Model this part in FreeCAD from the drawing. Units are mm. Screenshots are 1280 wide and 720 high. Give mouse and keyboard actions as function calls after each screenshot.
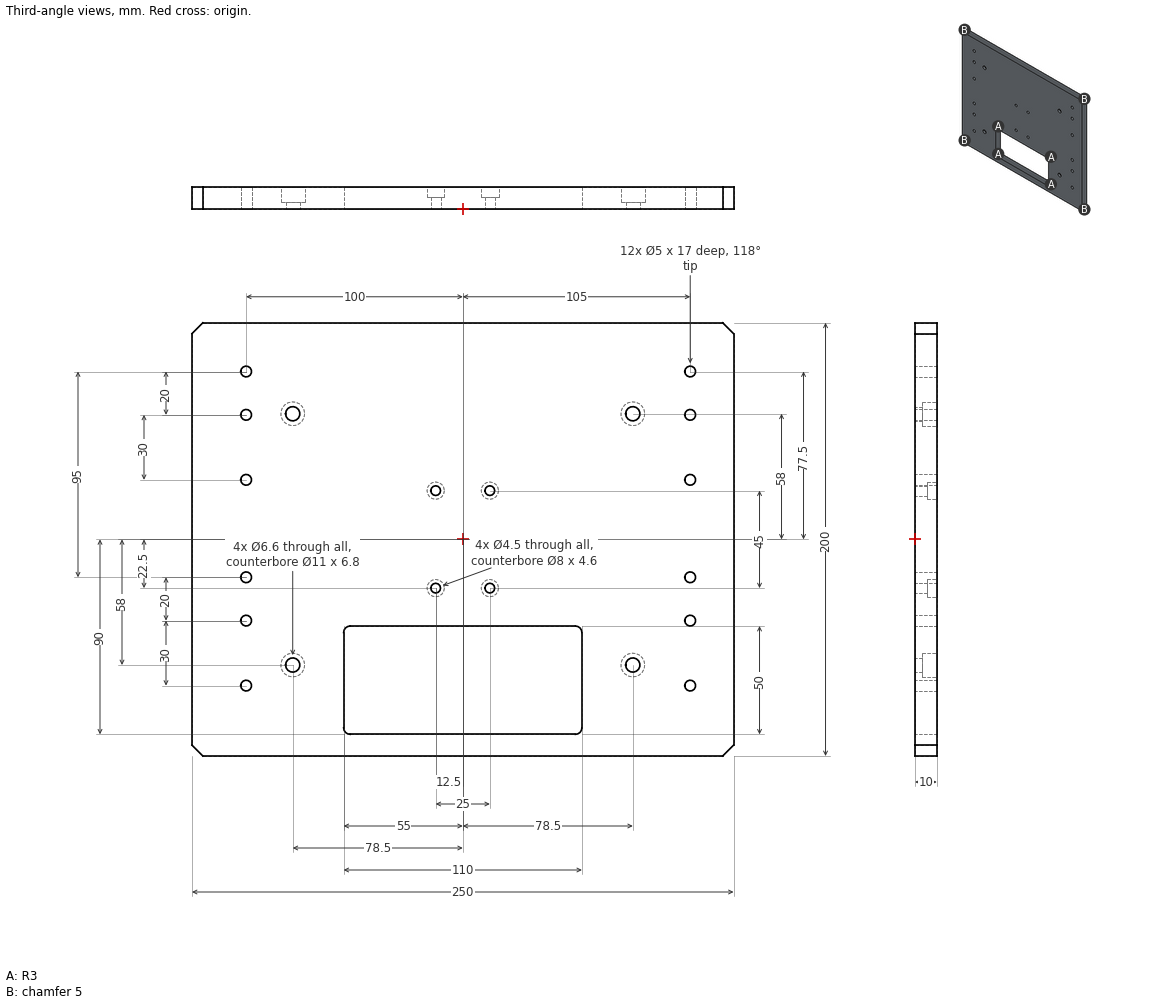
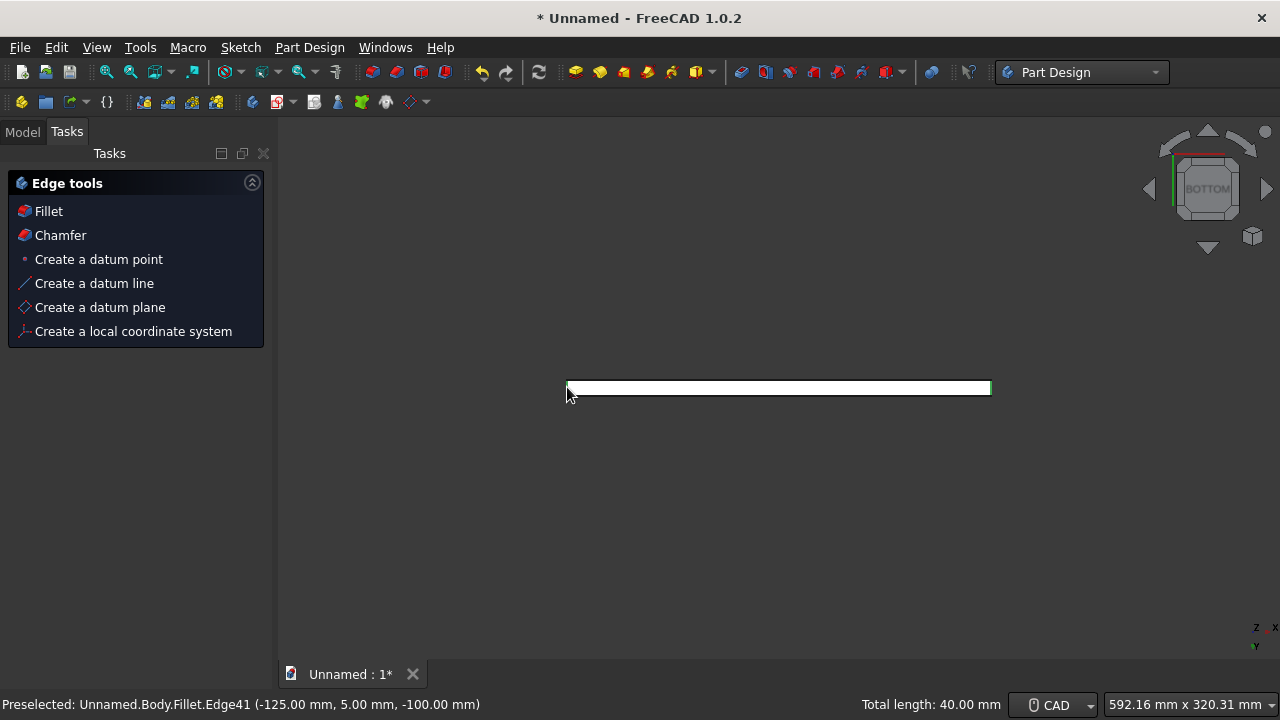
click(398, 72)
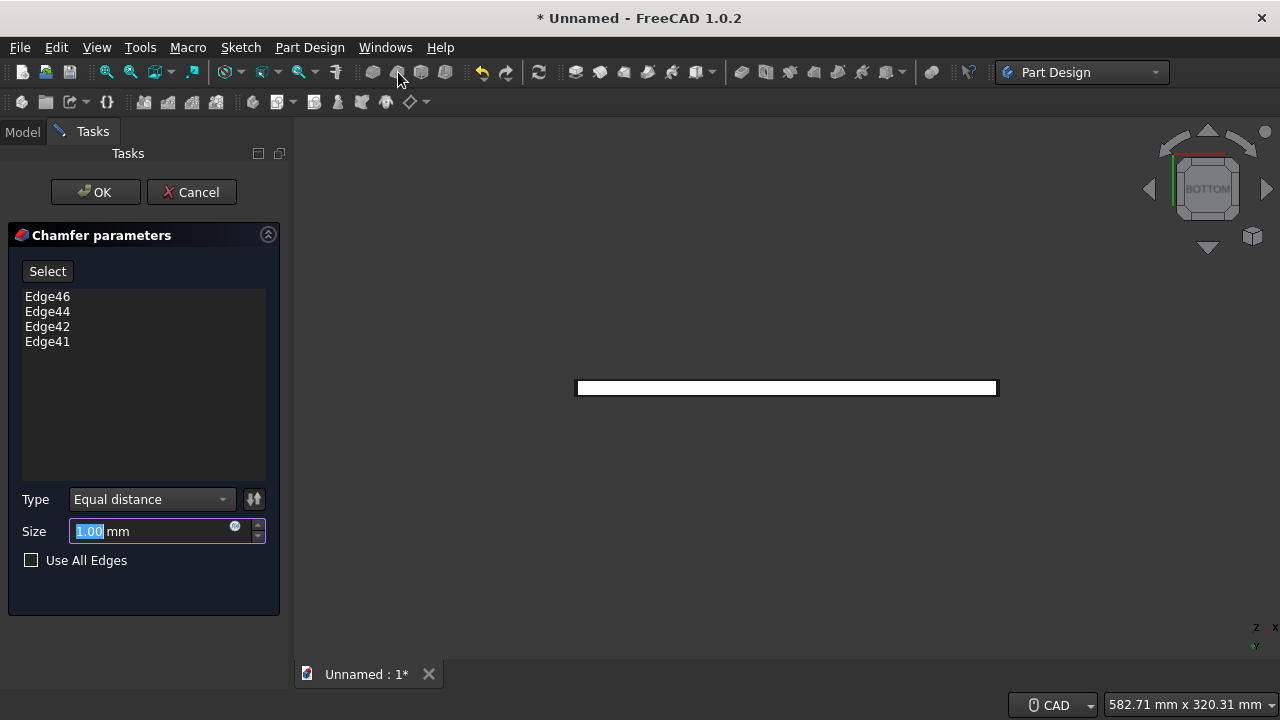
text(5)
key(Tab)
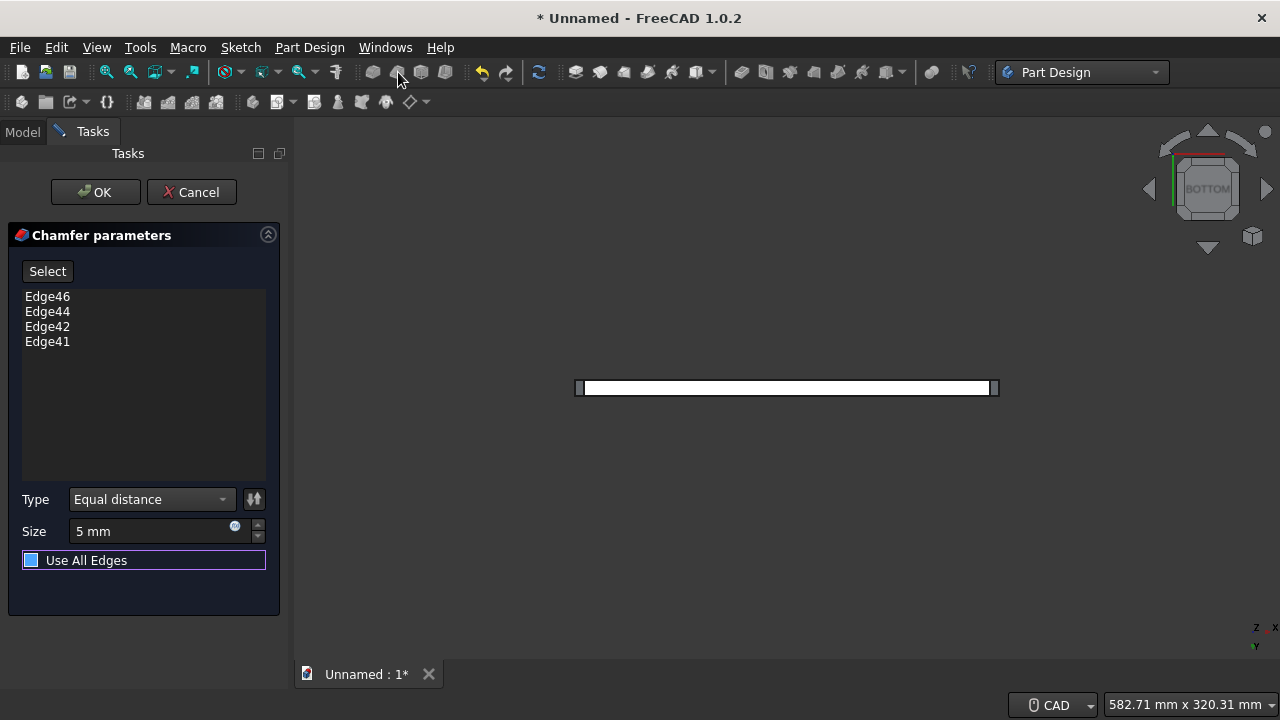
click(96, 192)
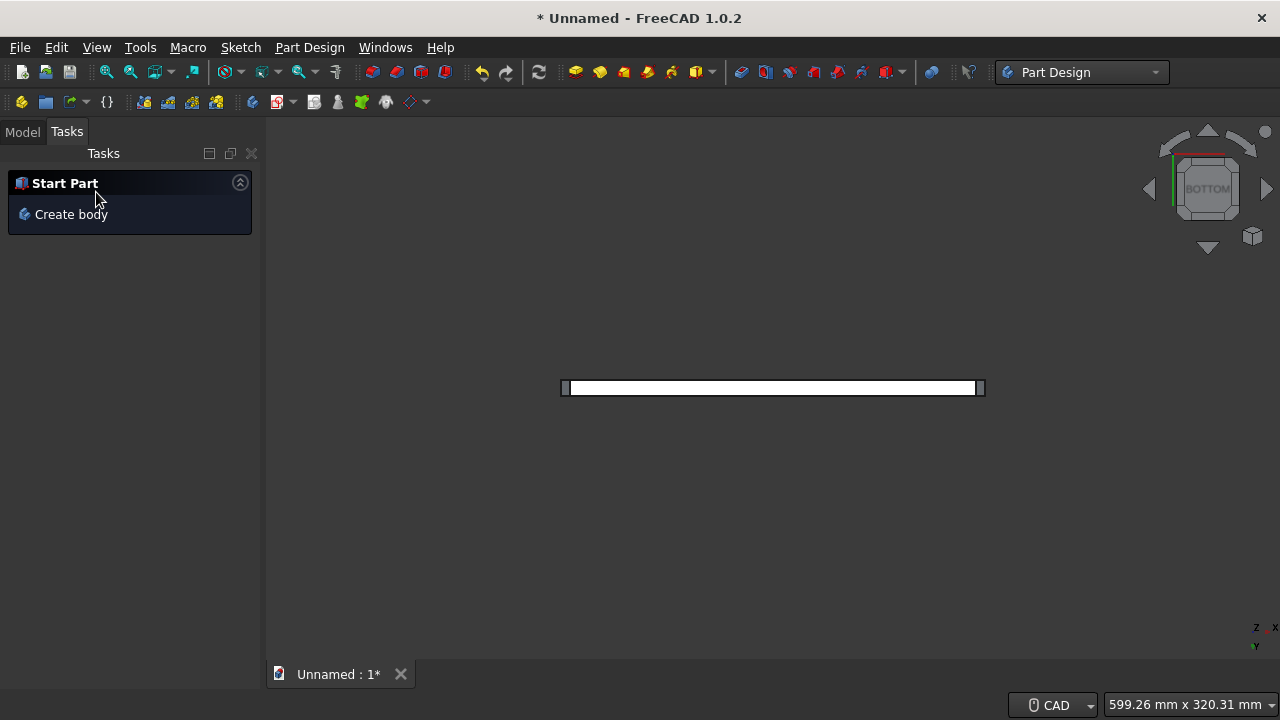
click(108, 72)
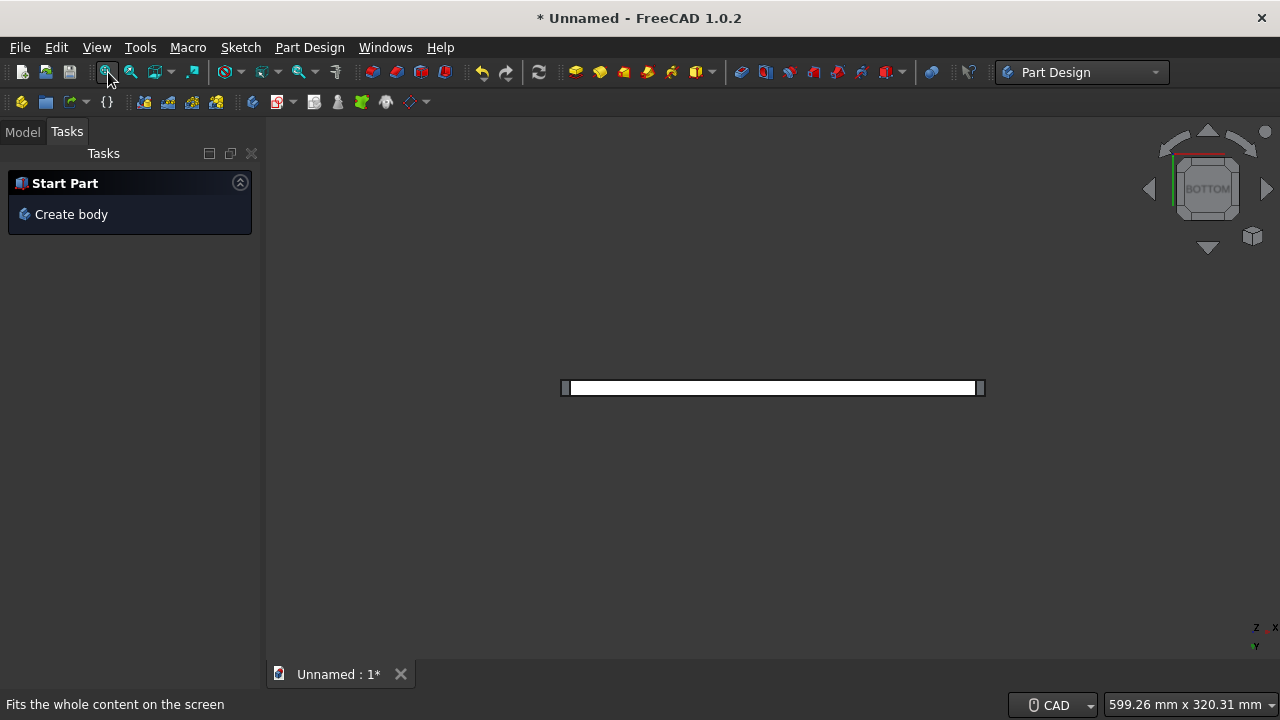
key(4)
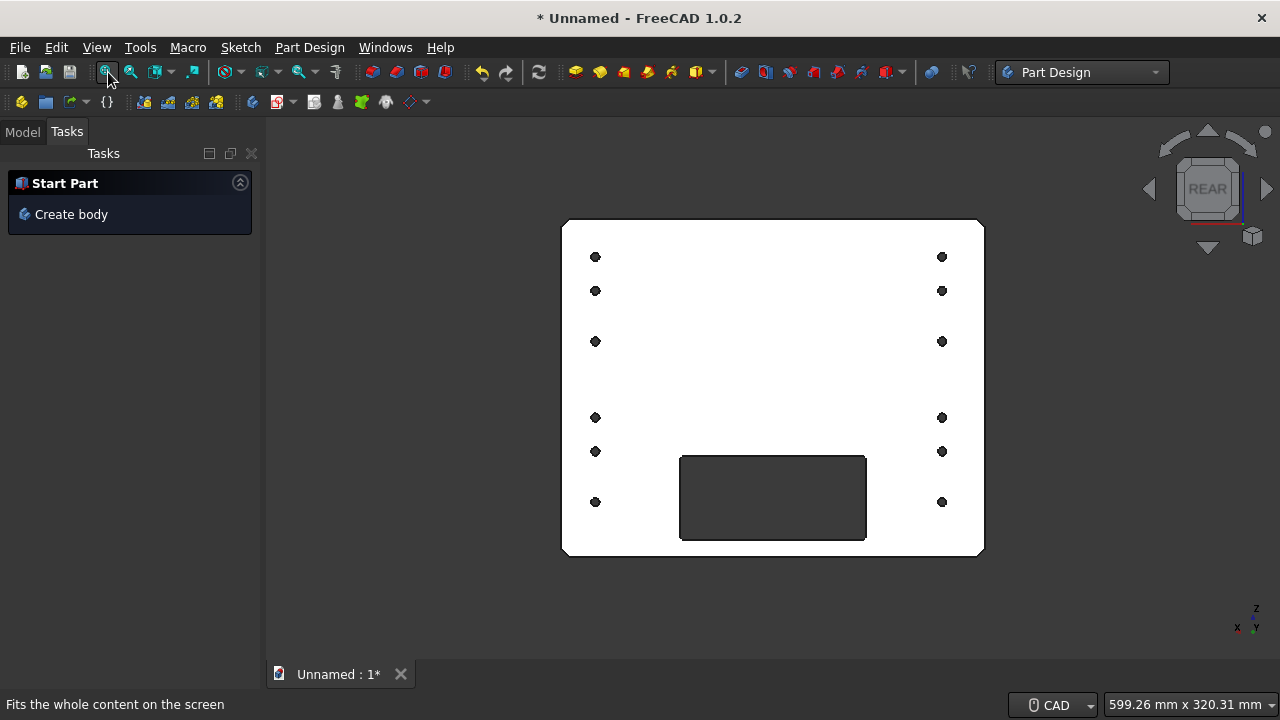
click(773, 339)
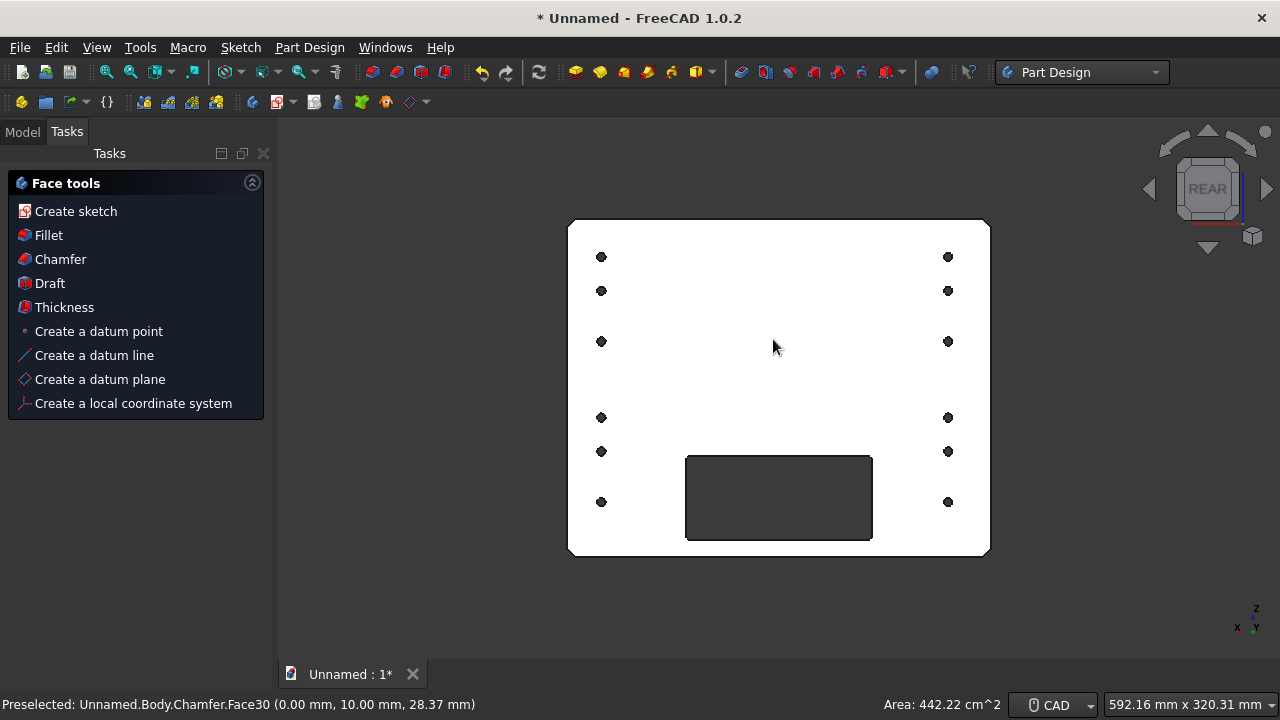
click(278, 102)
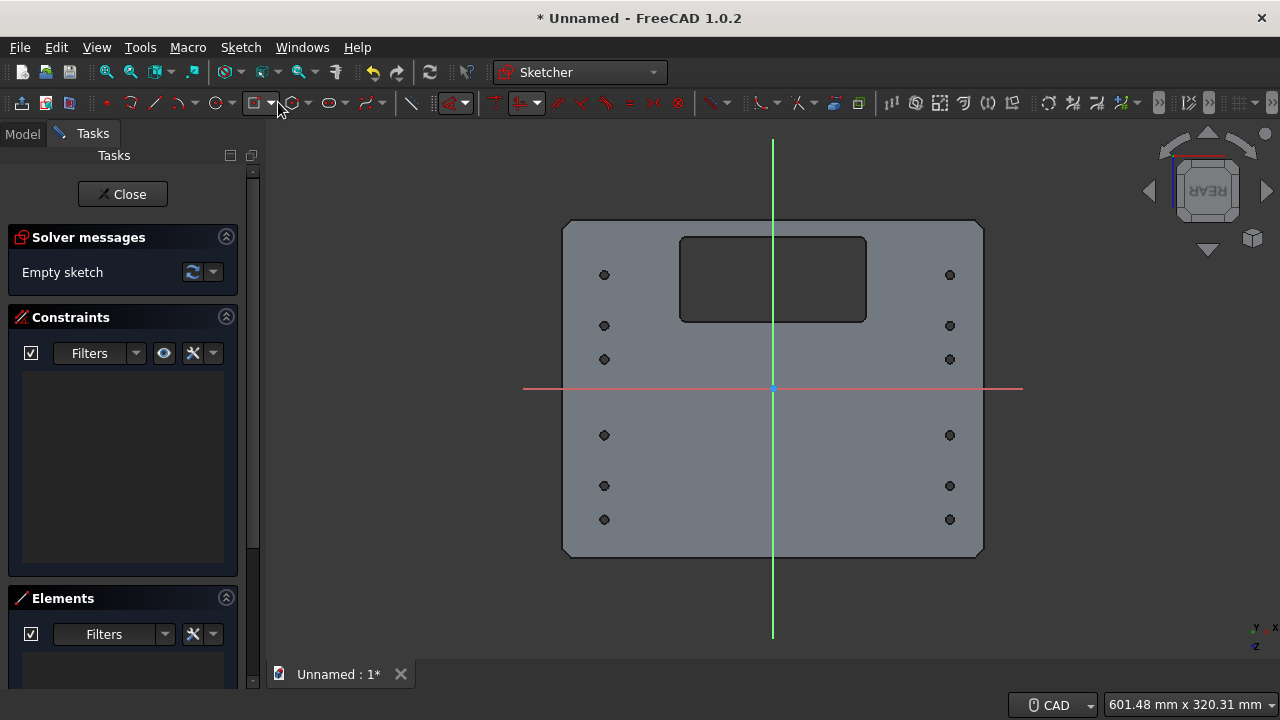
scroll(856, 389, up, 3)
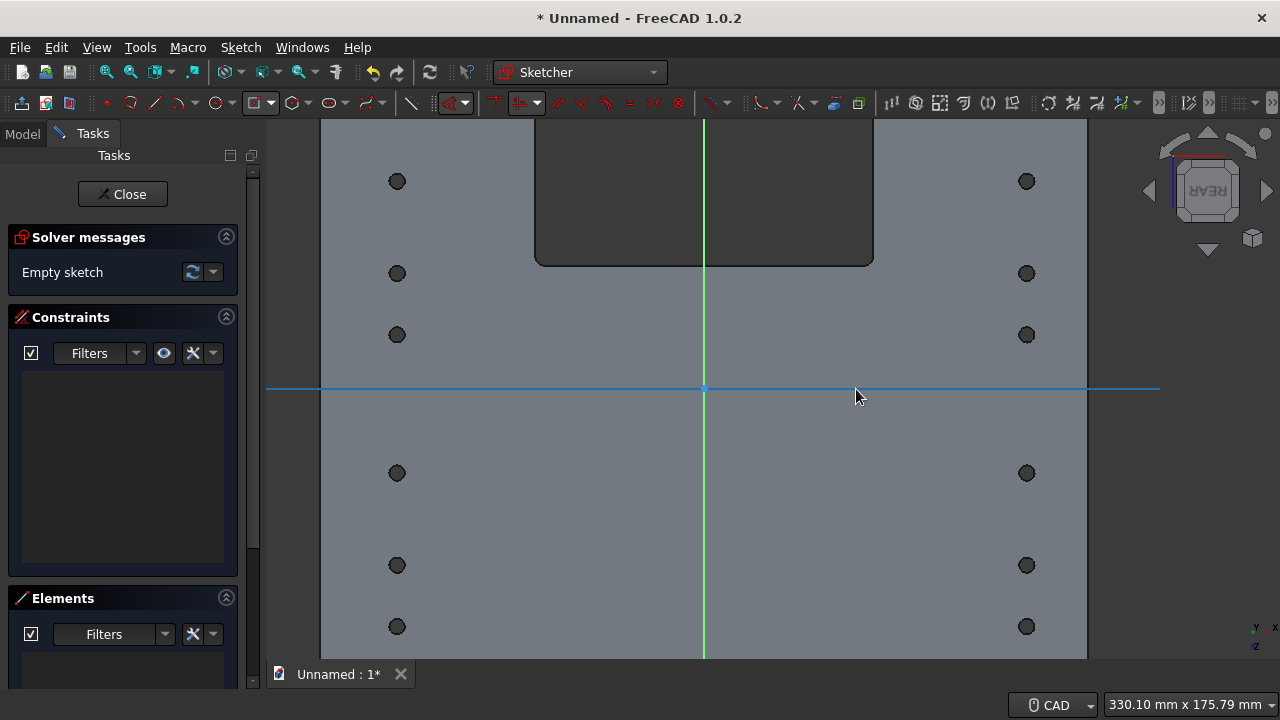
click(216, 104)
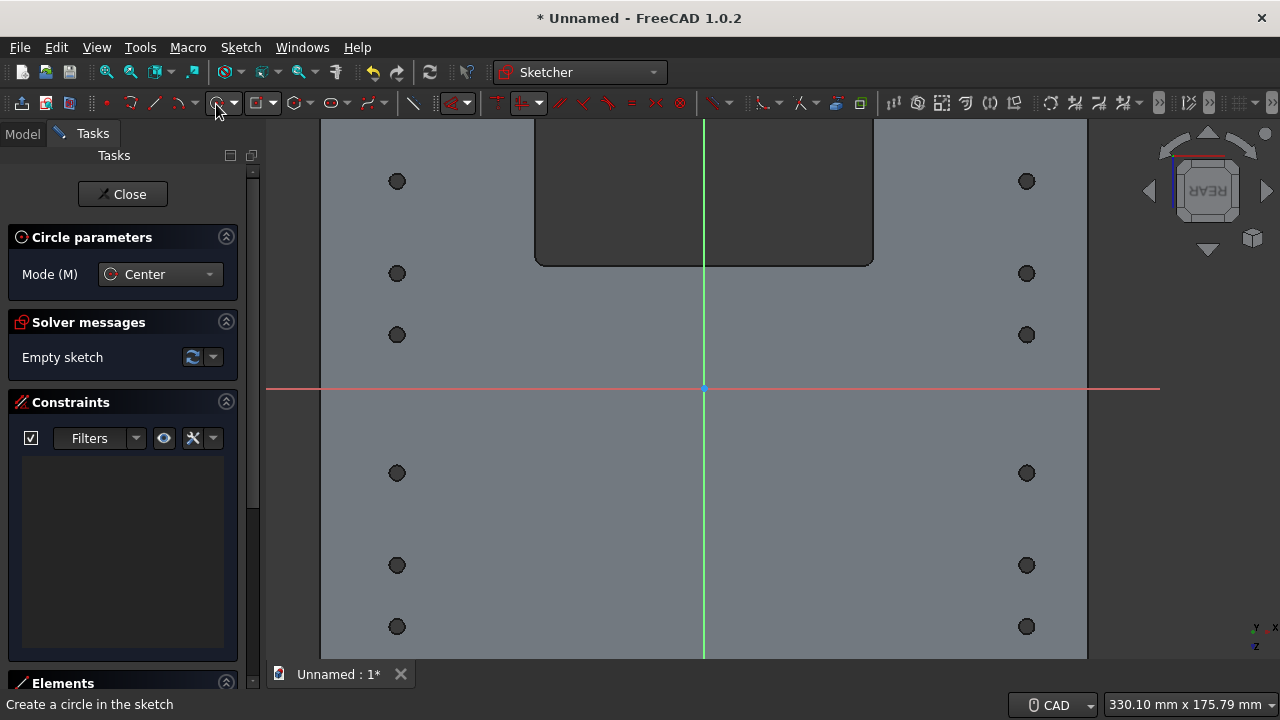
scroll(463, 210, up, 5)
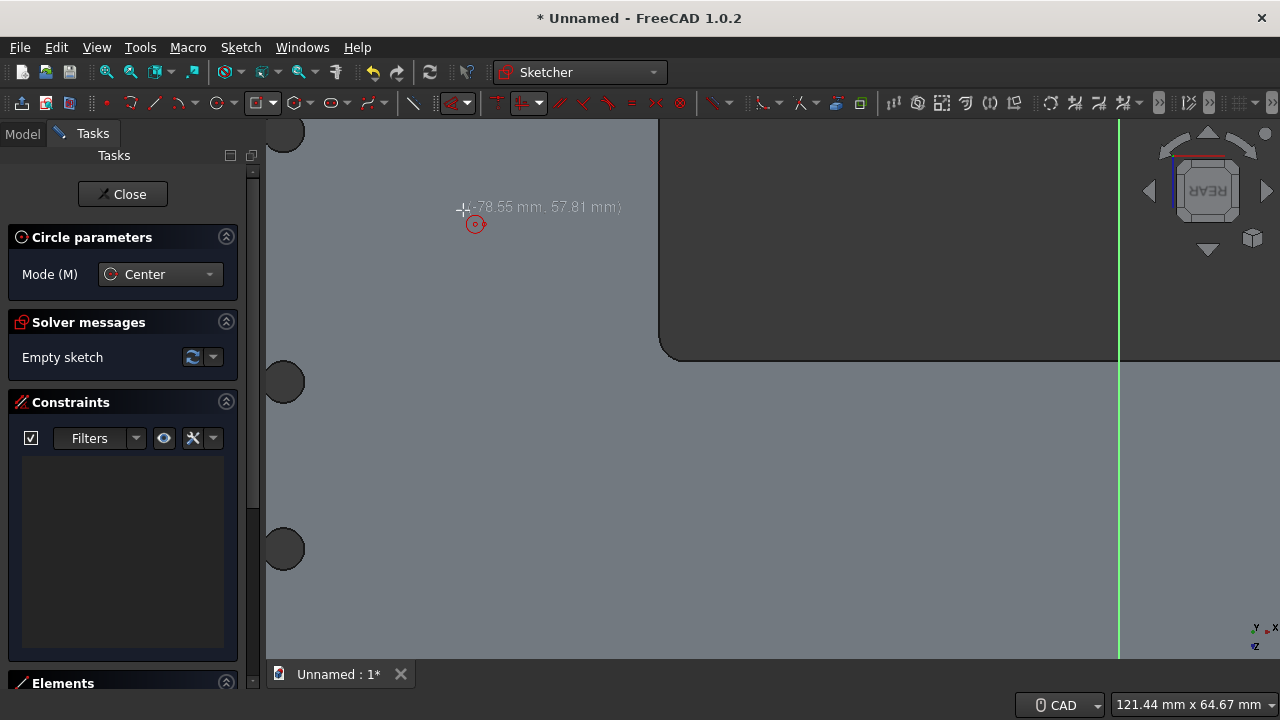
click(463, 211)
move(483, 191)